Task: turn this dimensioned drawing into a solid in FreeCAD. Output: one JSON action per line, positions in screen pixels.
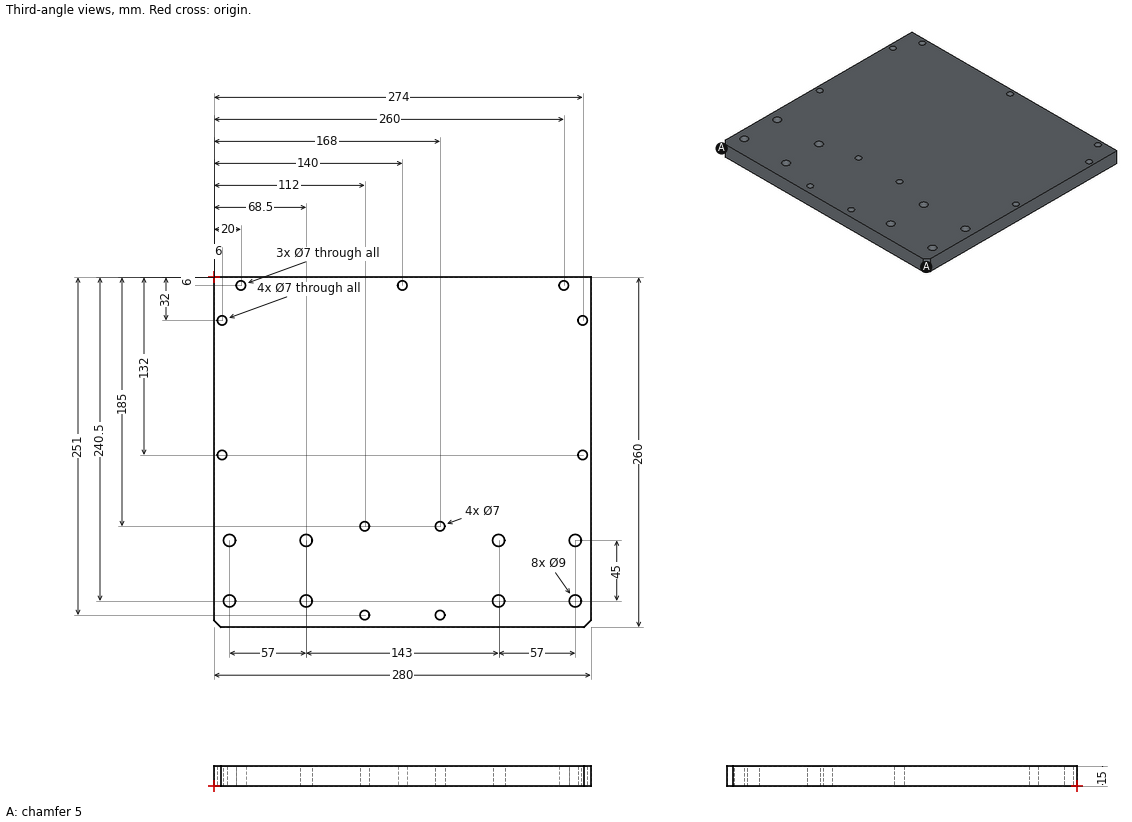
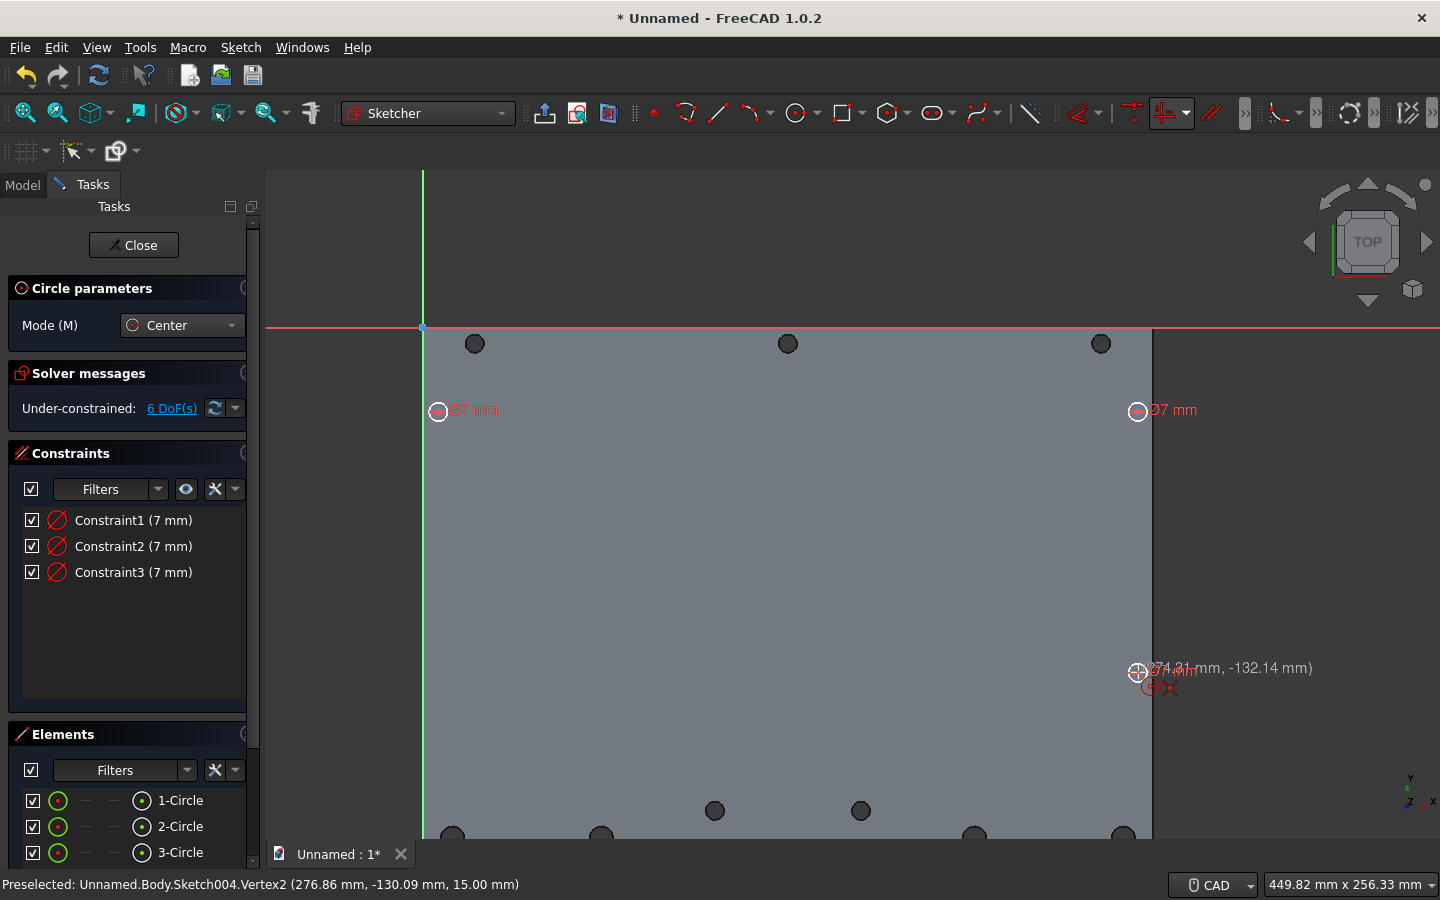
{"action": "scroll", "coordinate": [438, 672], "scroll_direction": "up", "scroll_amount": 5}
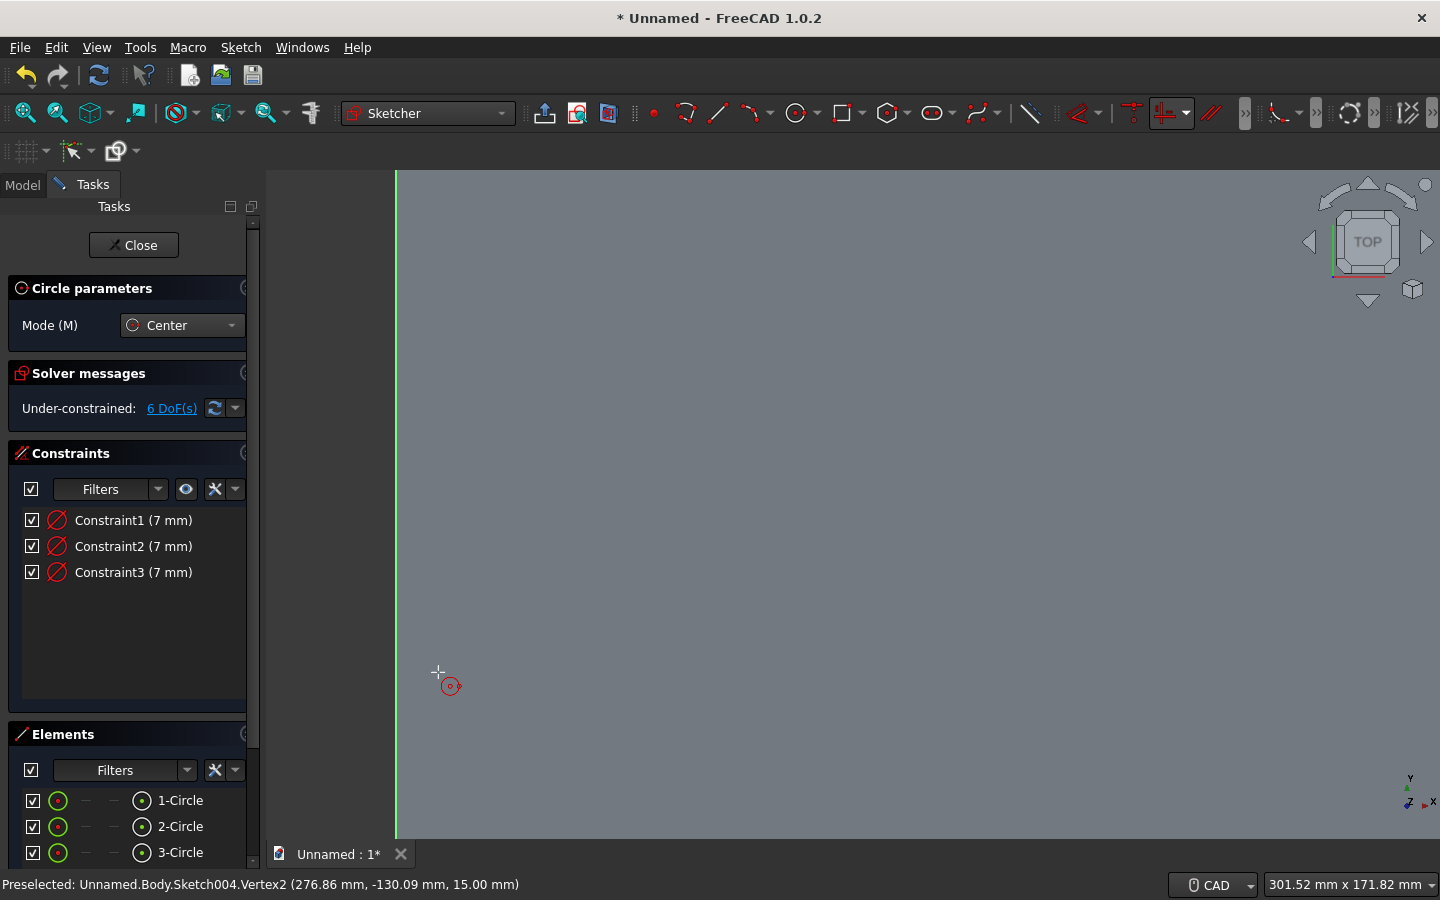
{"action": "left_click", "coordinate": [438, 672]}
{"action": "mouse_move", "coordinate": [456, 654]}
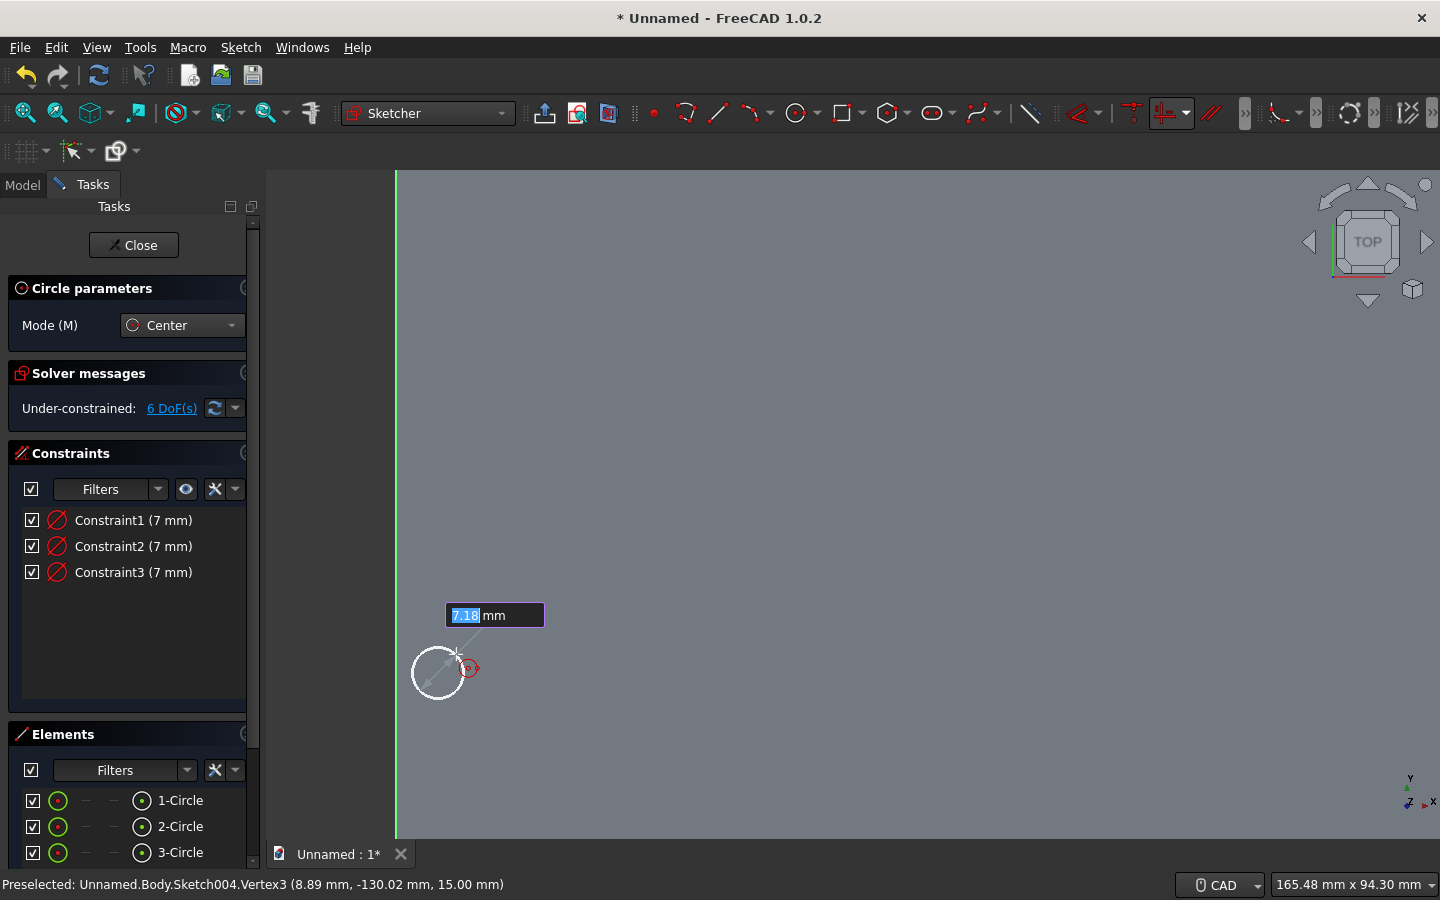
{"action": "type", "text": "7"}
{"action": "key", "text": "Return"}
{"action": "key", "text": "Escape"}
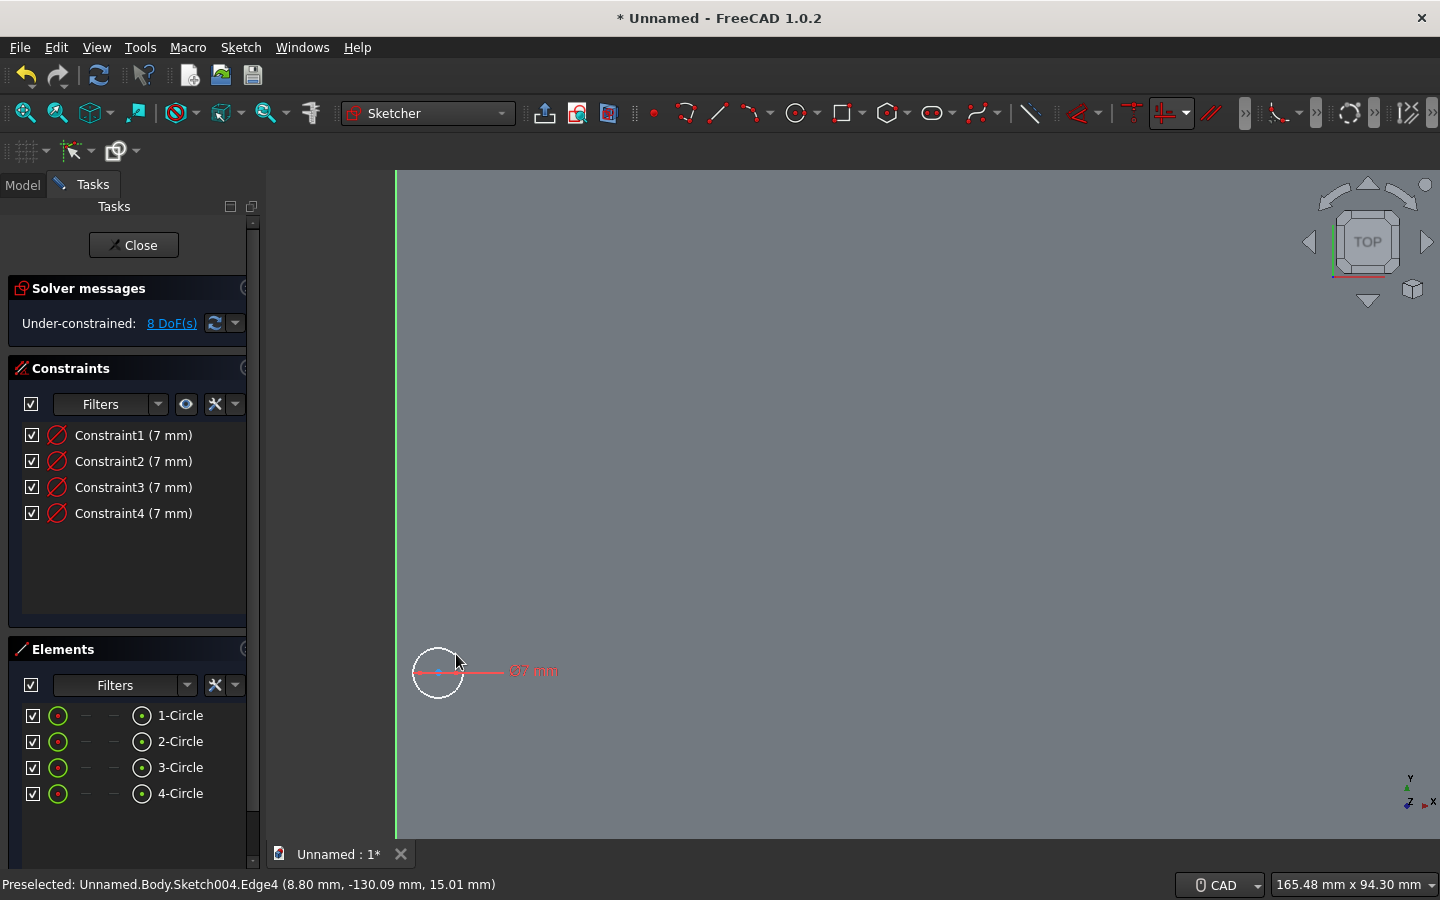
{"action": "scroll", "coordinate": [438, 672], "scroll_direction": "down", "scroll_amount": 5}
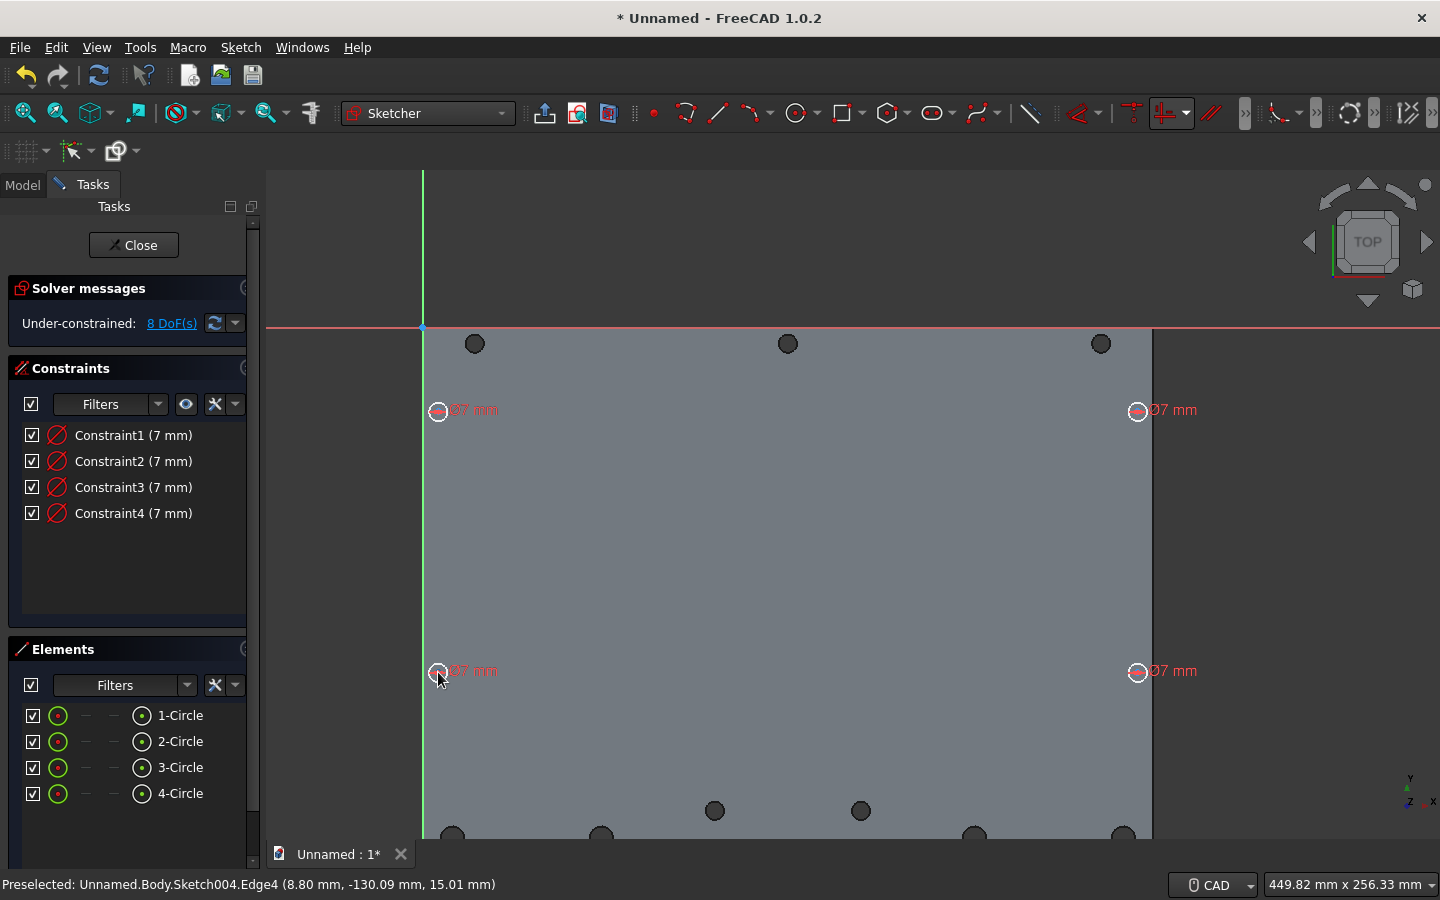
{"action": "left_click", "coordinate": [438, 412]}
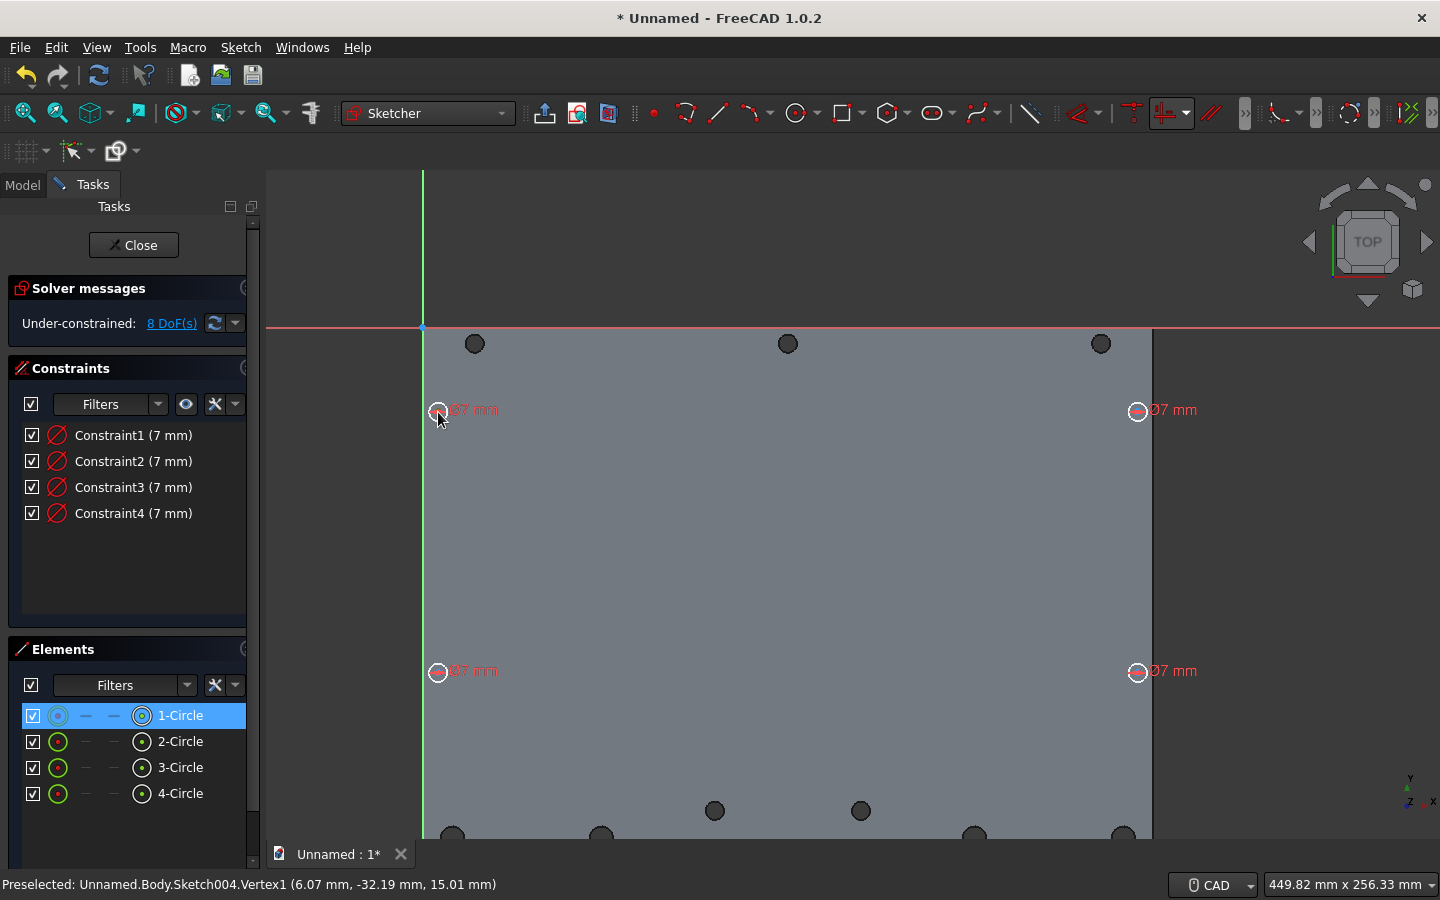
{"action": "left_click", "coordinate": [1138, 412]}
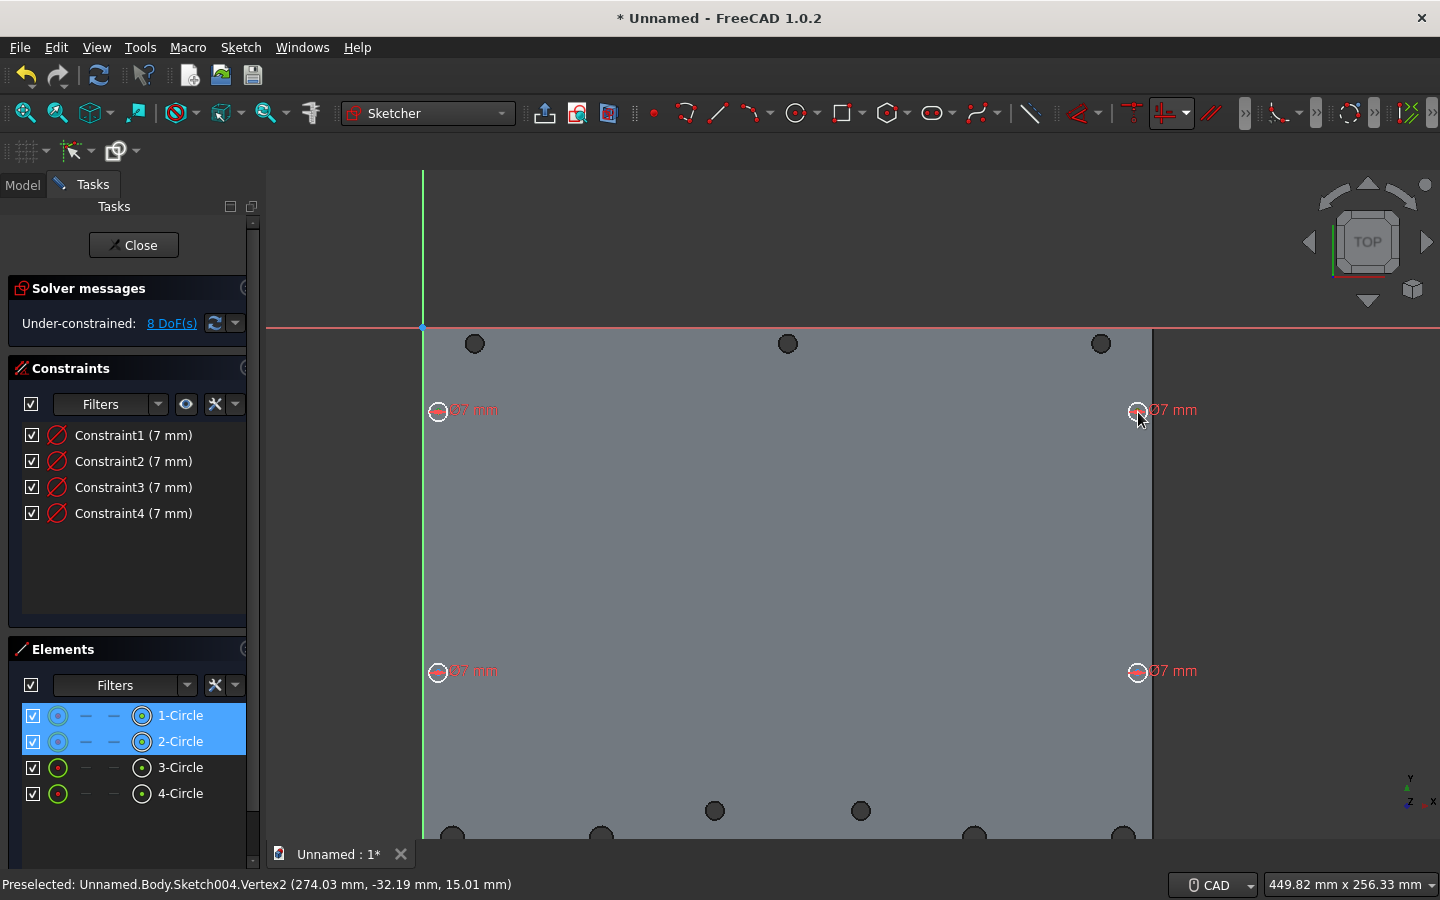
{"action": "key", "text": "h"}